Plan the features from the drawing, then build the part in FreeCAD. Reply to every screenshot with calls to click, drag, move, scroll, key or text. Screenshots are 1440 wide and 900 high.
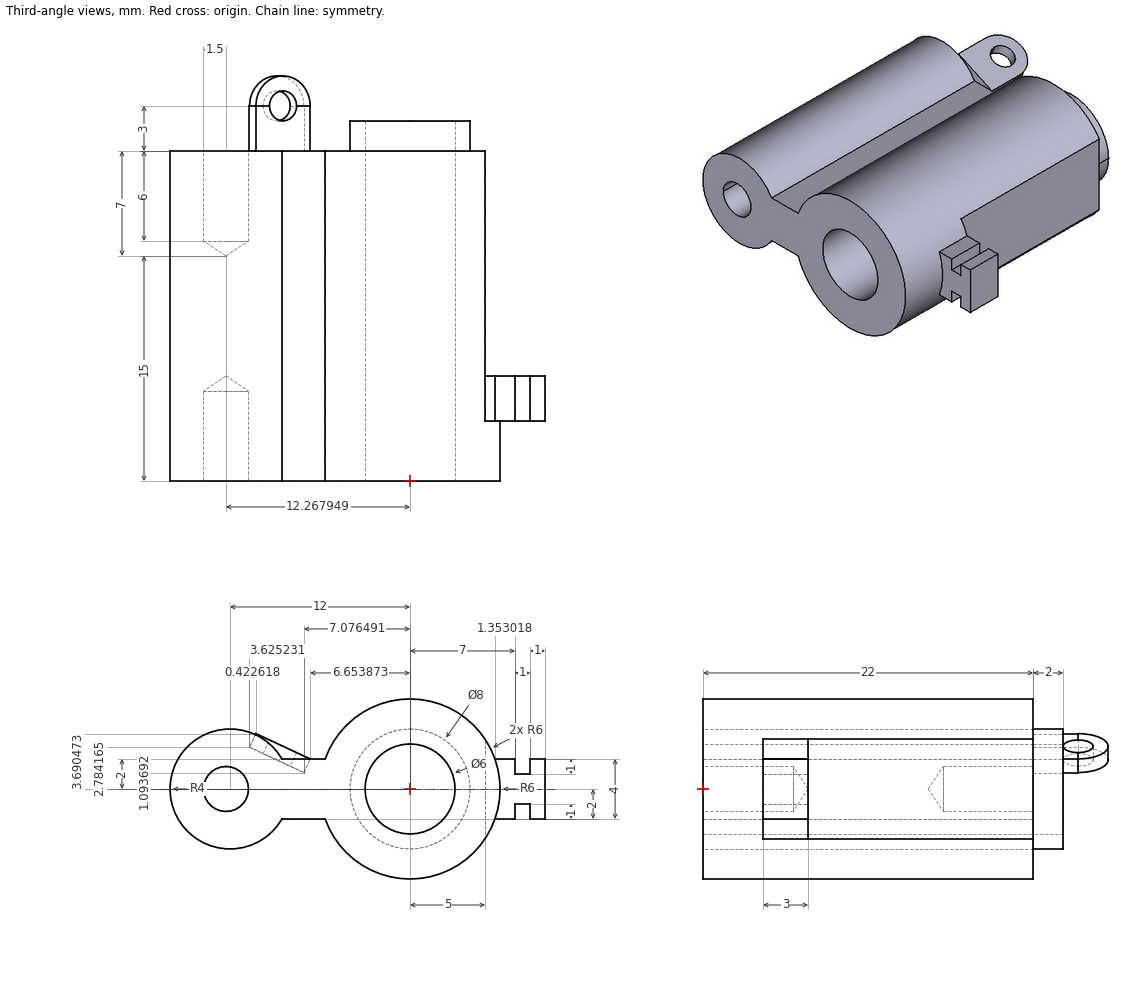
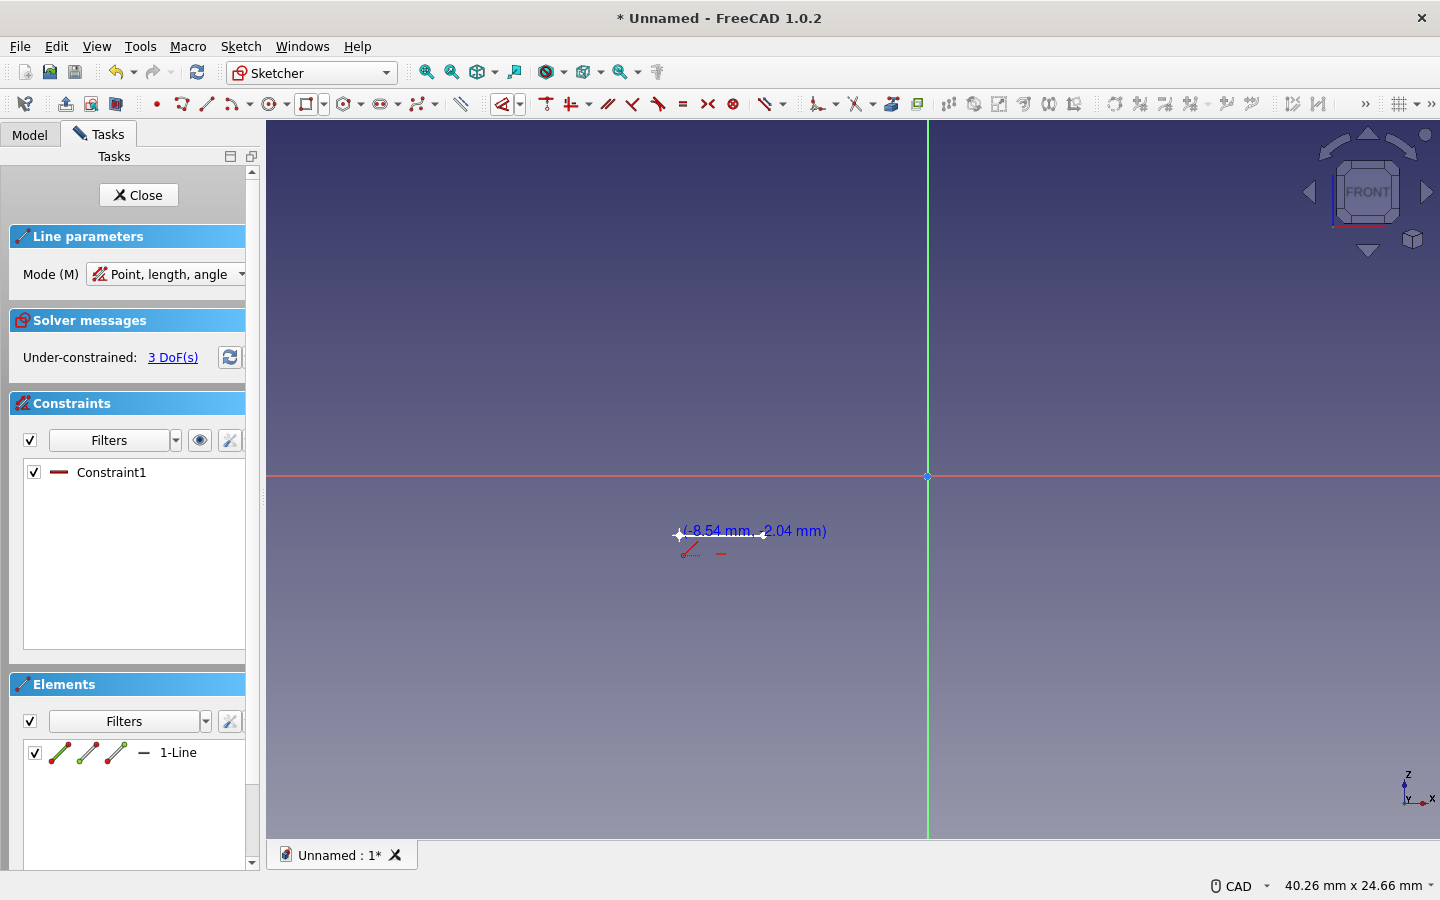
click(679, 418)
click(763, 418)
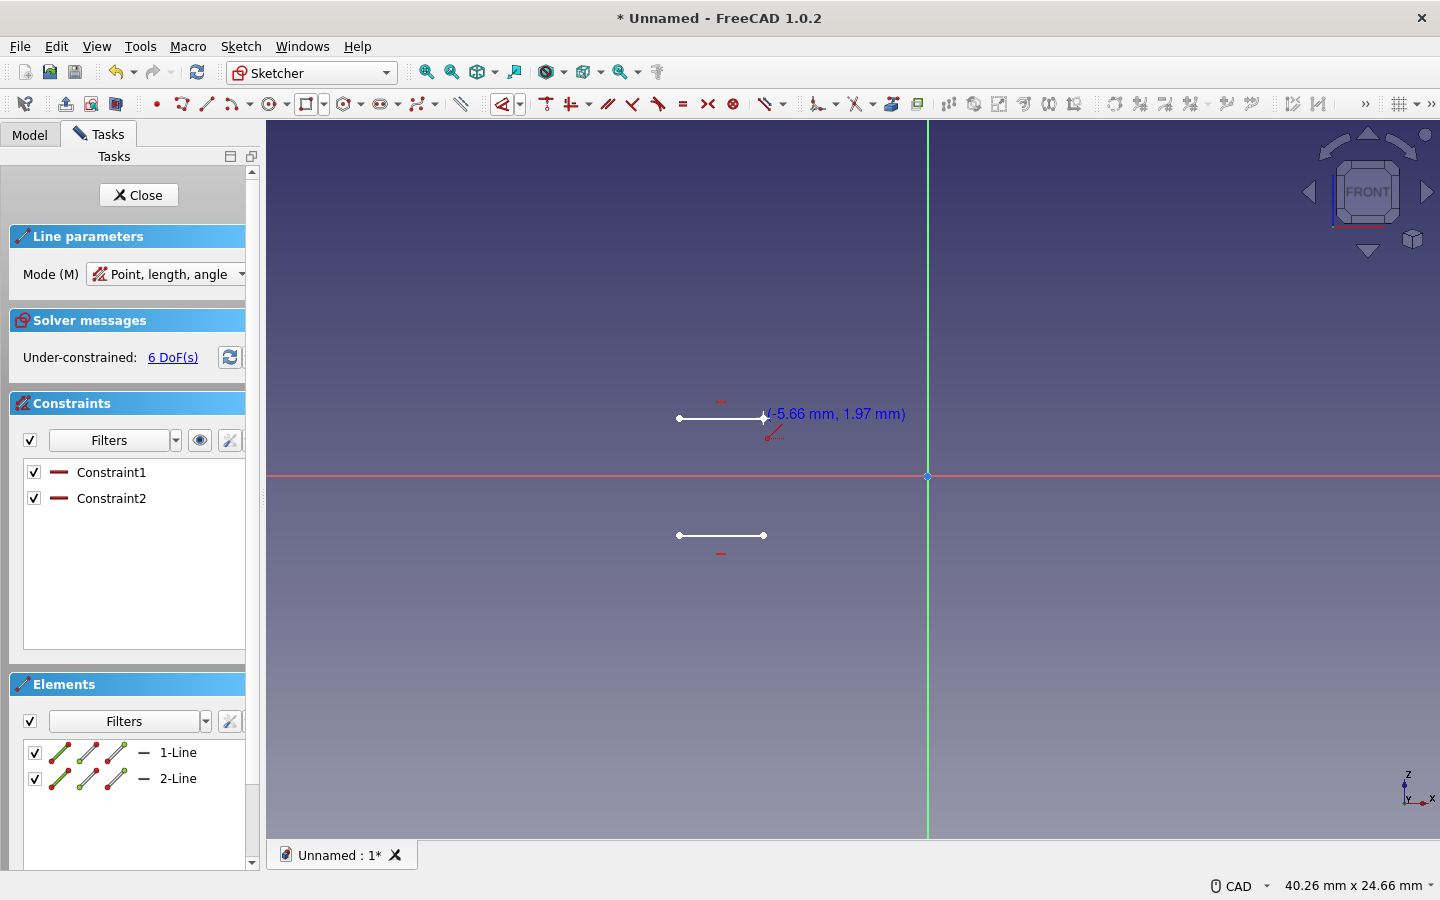
click(250, 104)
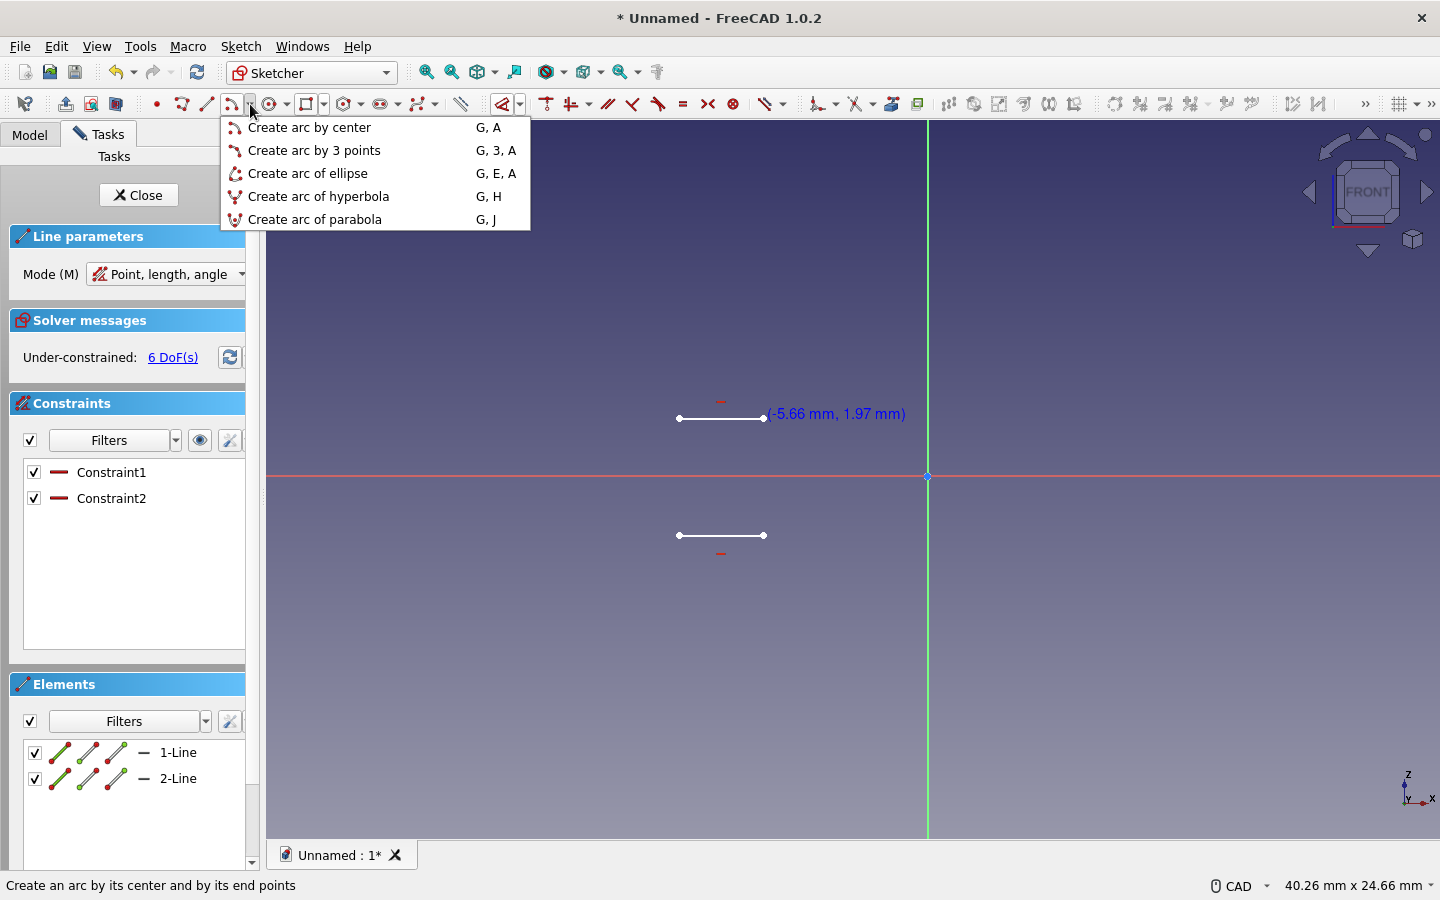
click(376, 150)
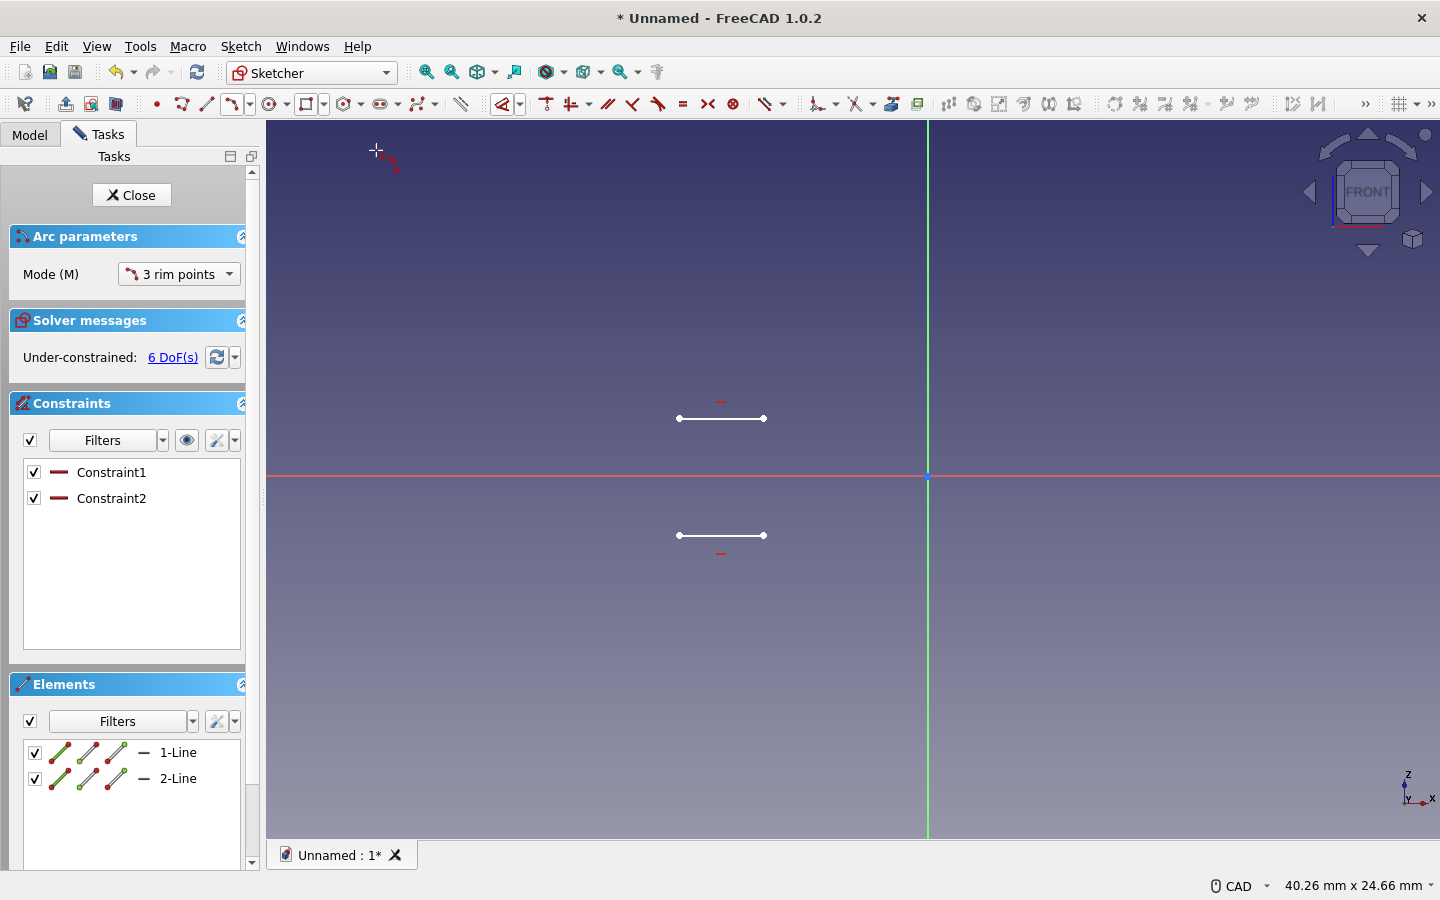
click(679, 536)
click(679, 419)
click(477, 418)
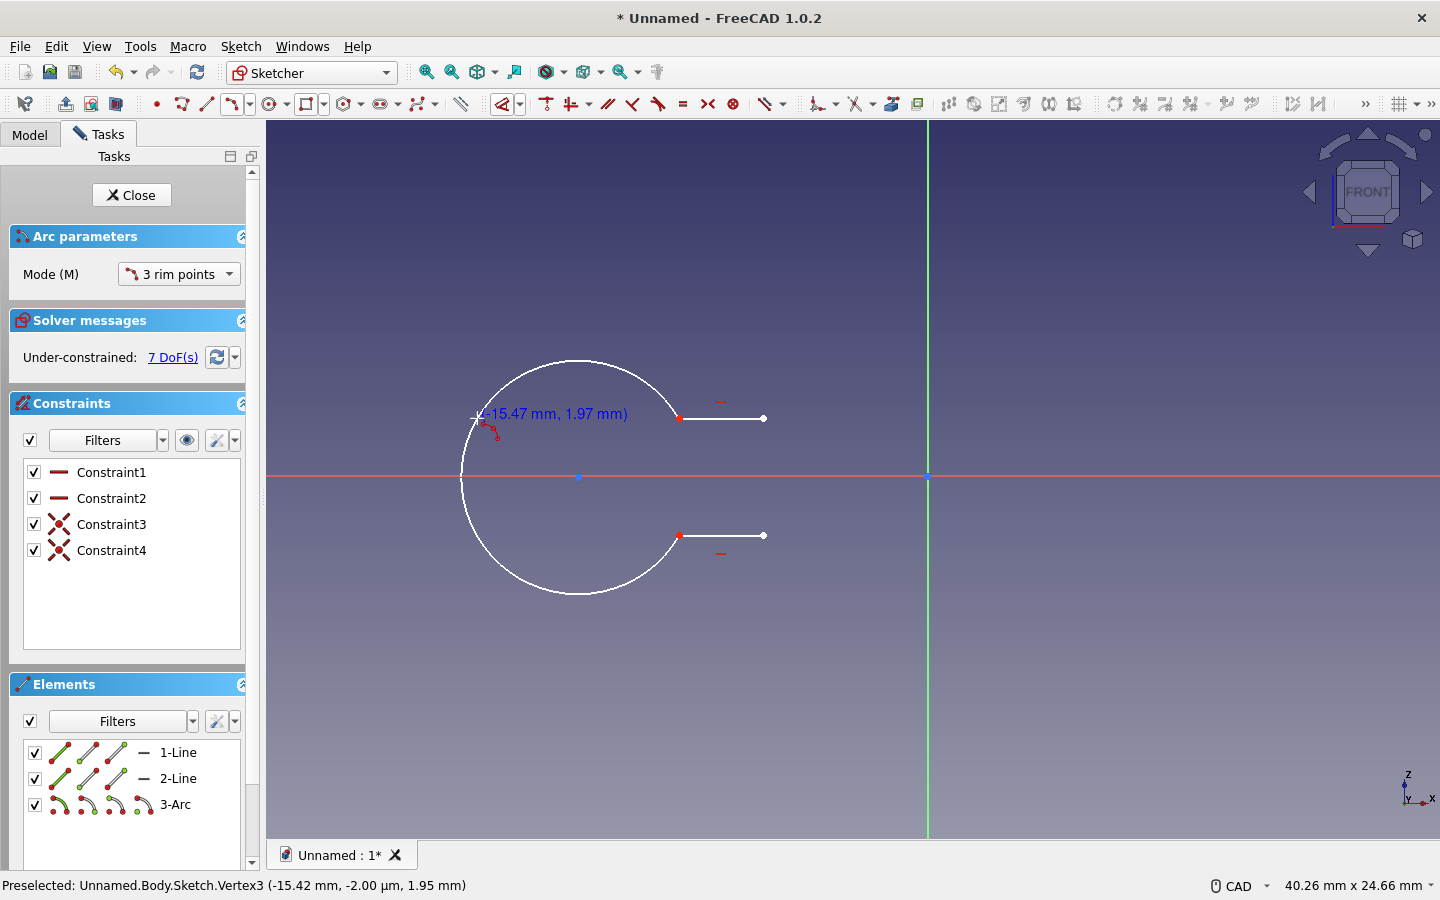
click(763, 419)
click(763, 536)
click(1076, 569)
key(Escape)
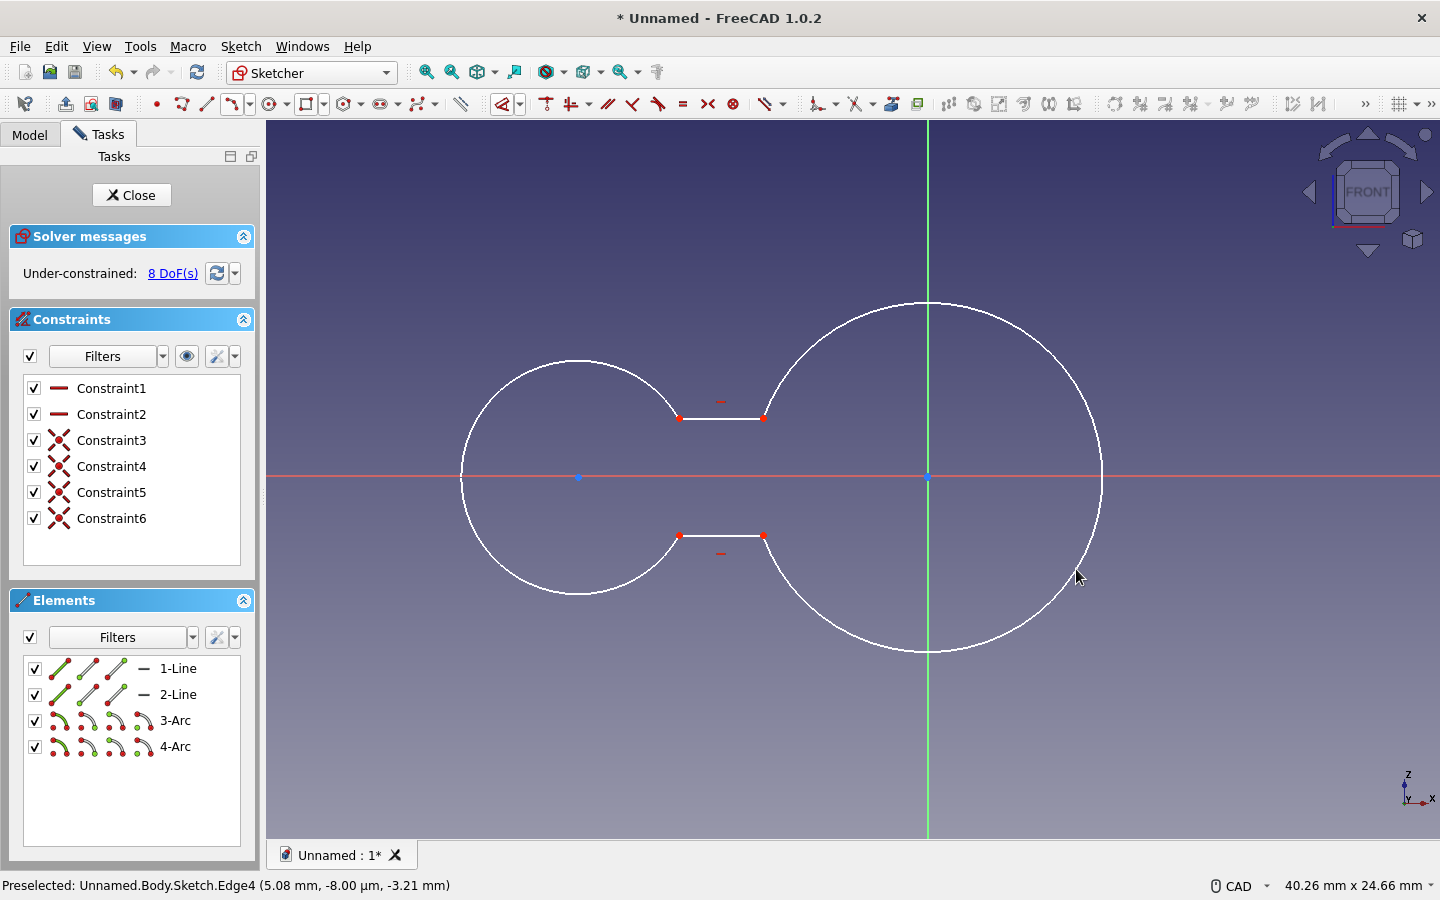
drag(918, 466, 938, 487)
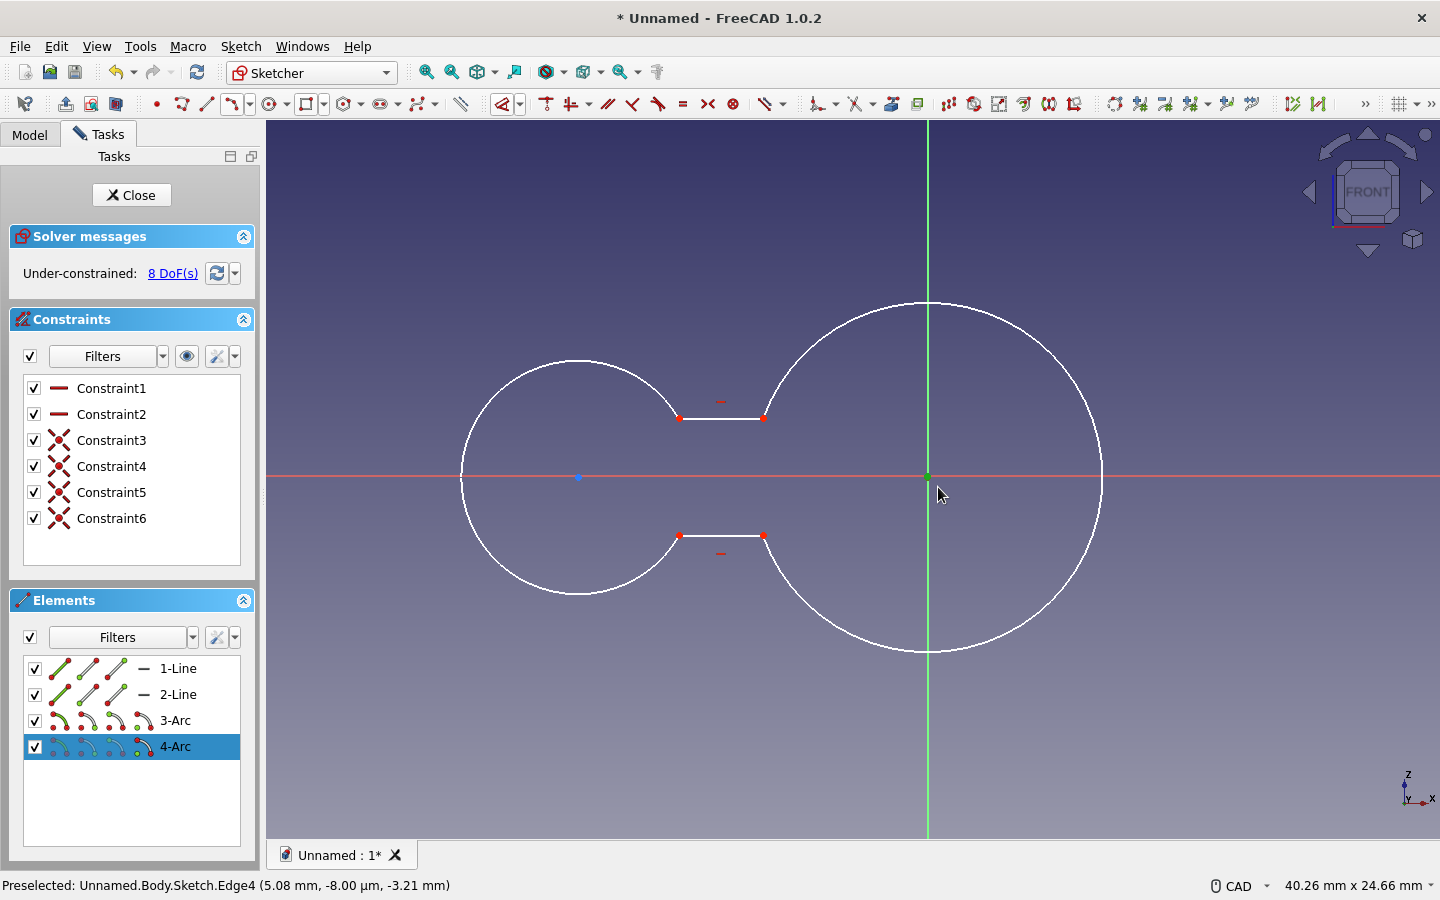
click(546, 104)